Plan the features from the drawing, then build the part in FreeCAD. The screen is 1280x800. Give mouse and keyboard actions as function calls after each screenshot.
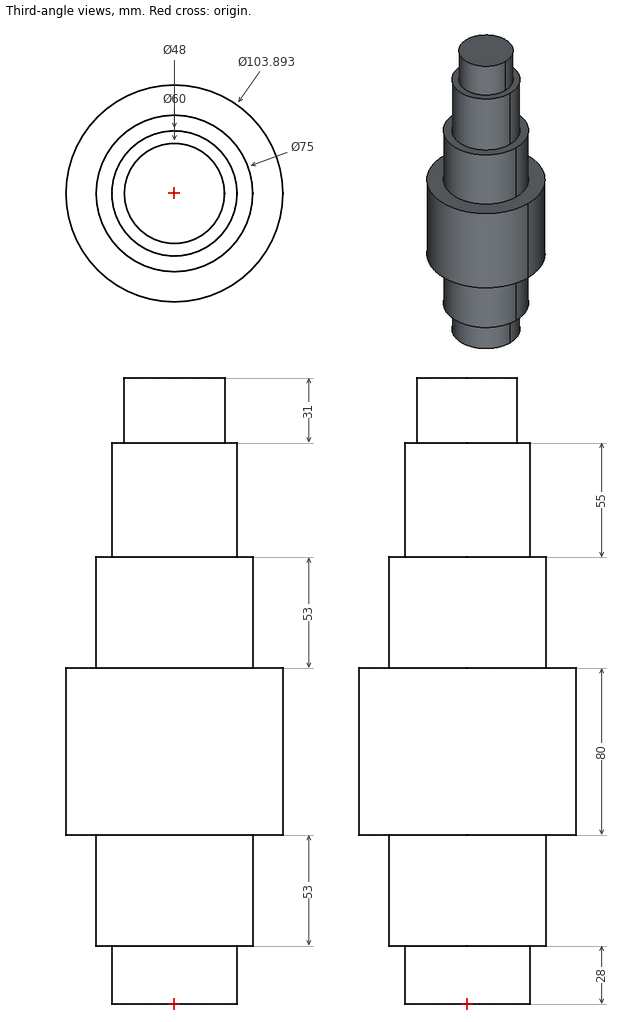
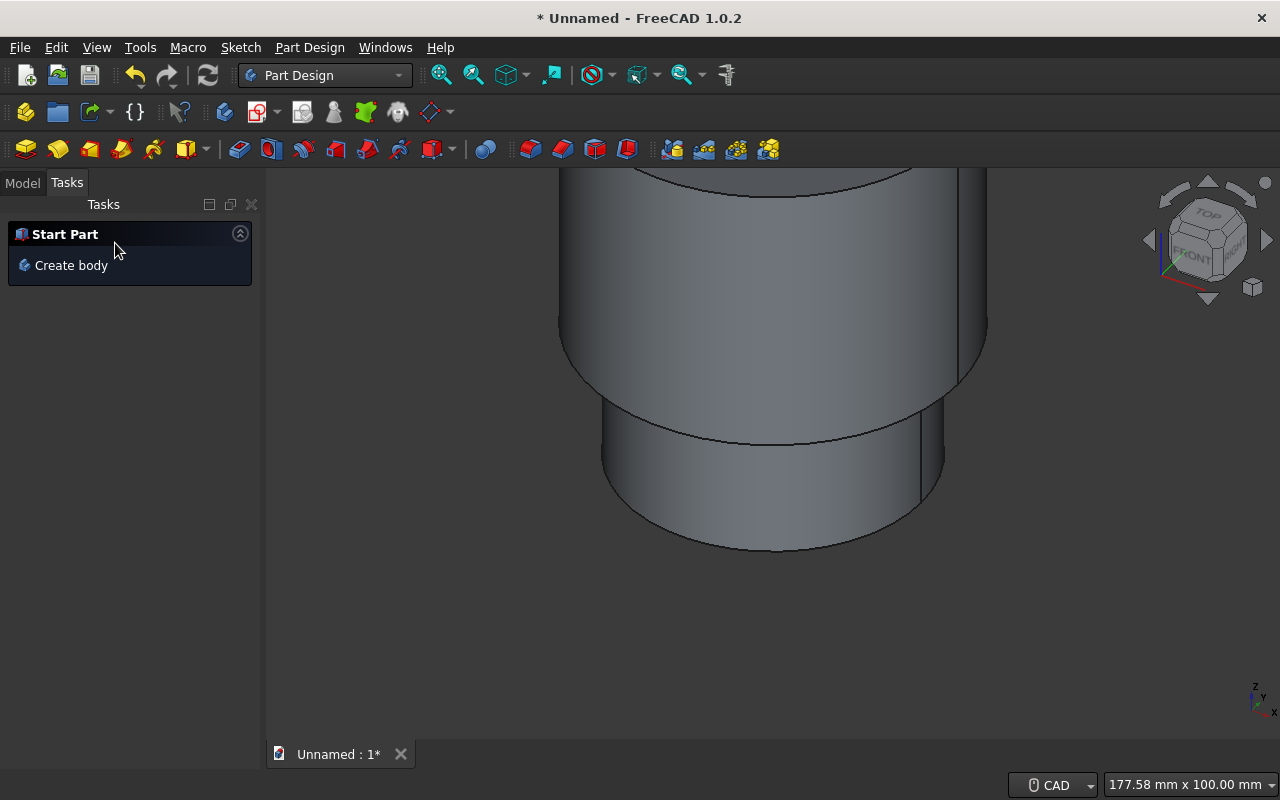
click(442, 76)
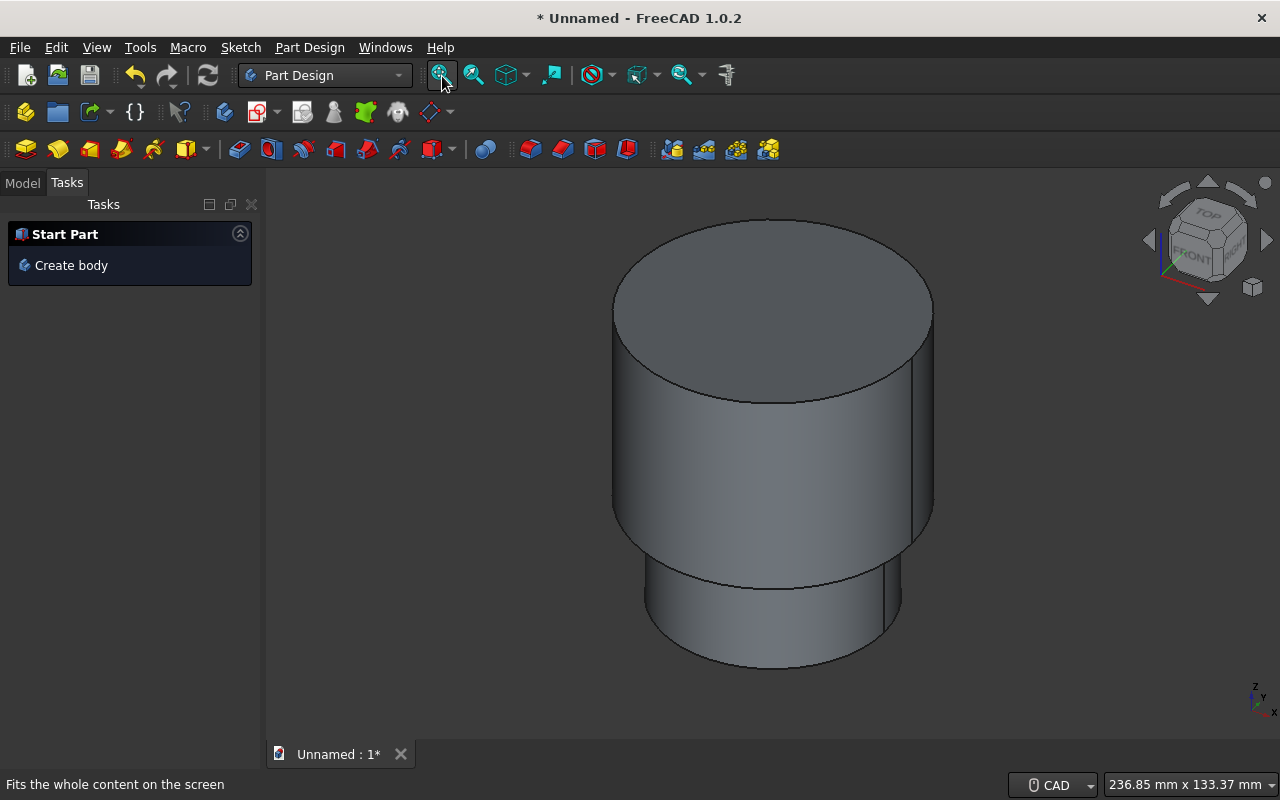
click(773, 310)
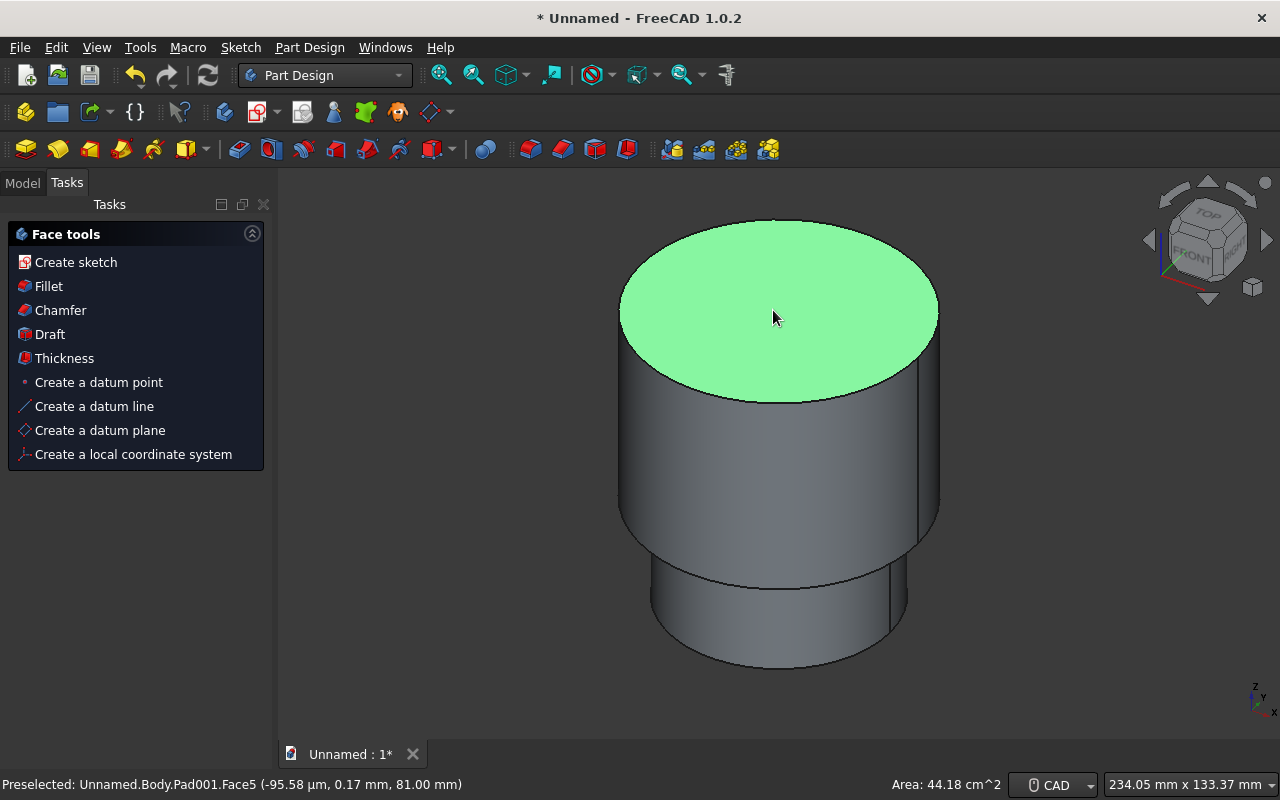
click(258, 112)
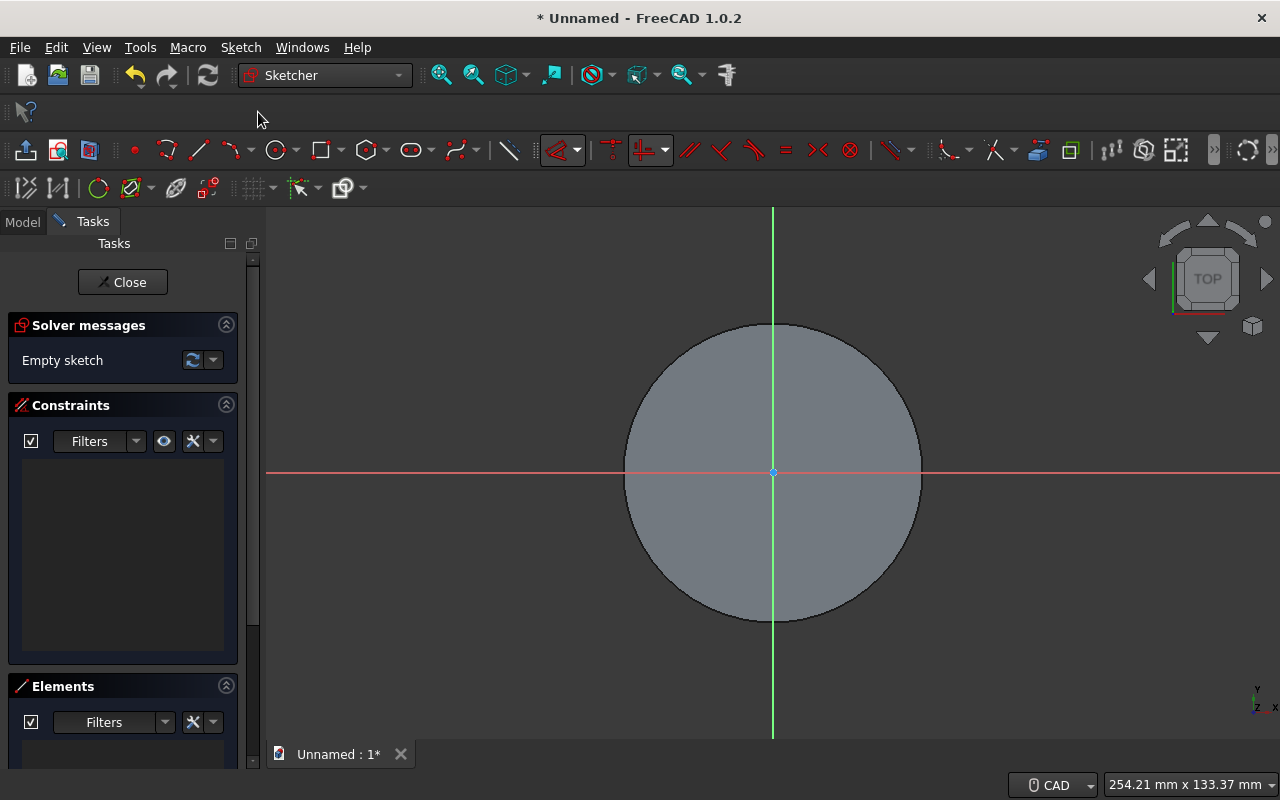
click(276, 150)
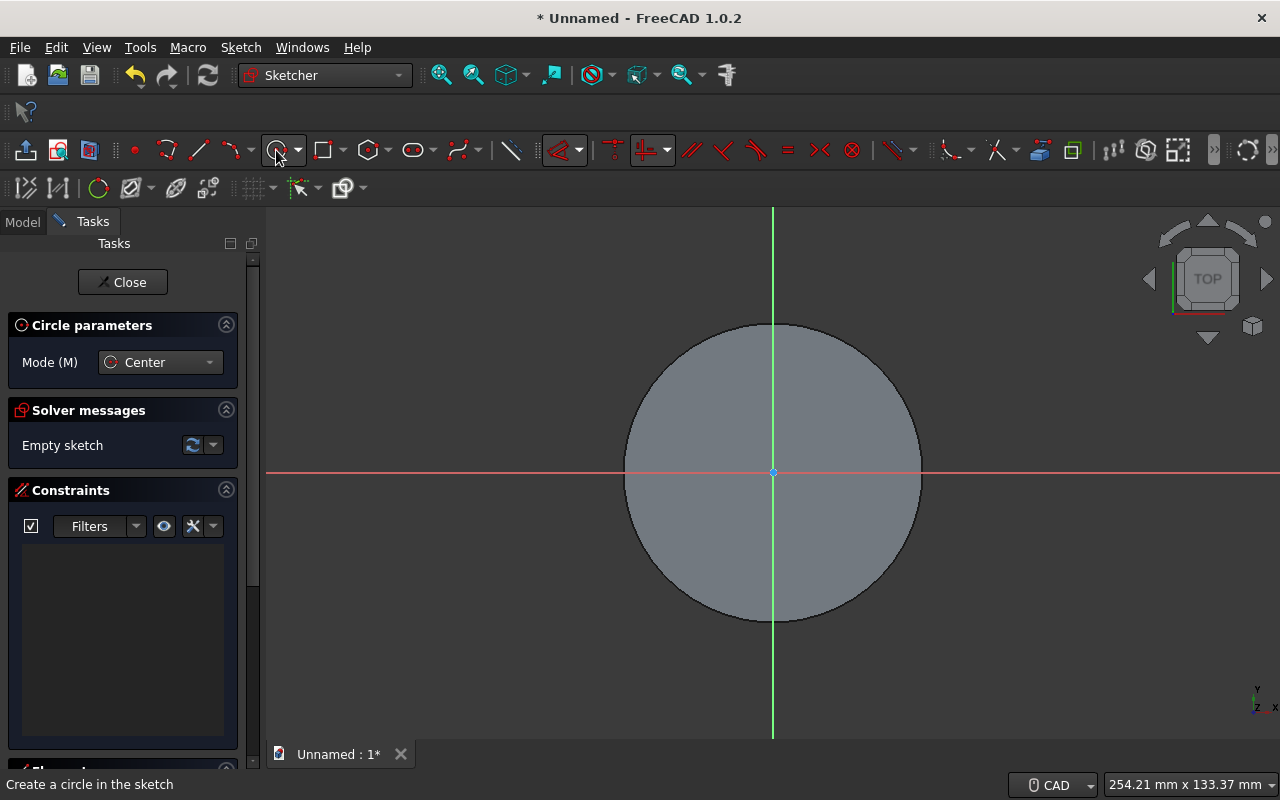
click(773, 473)
move(920, 326)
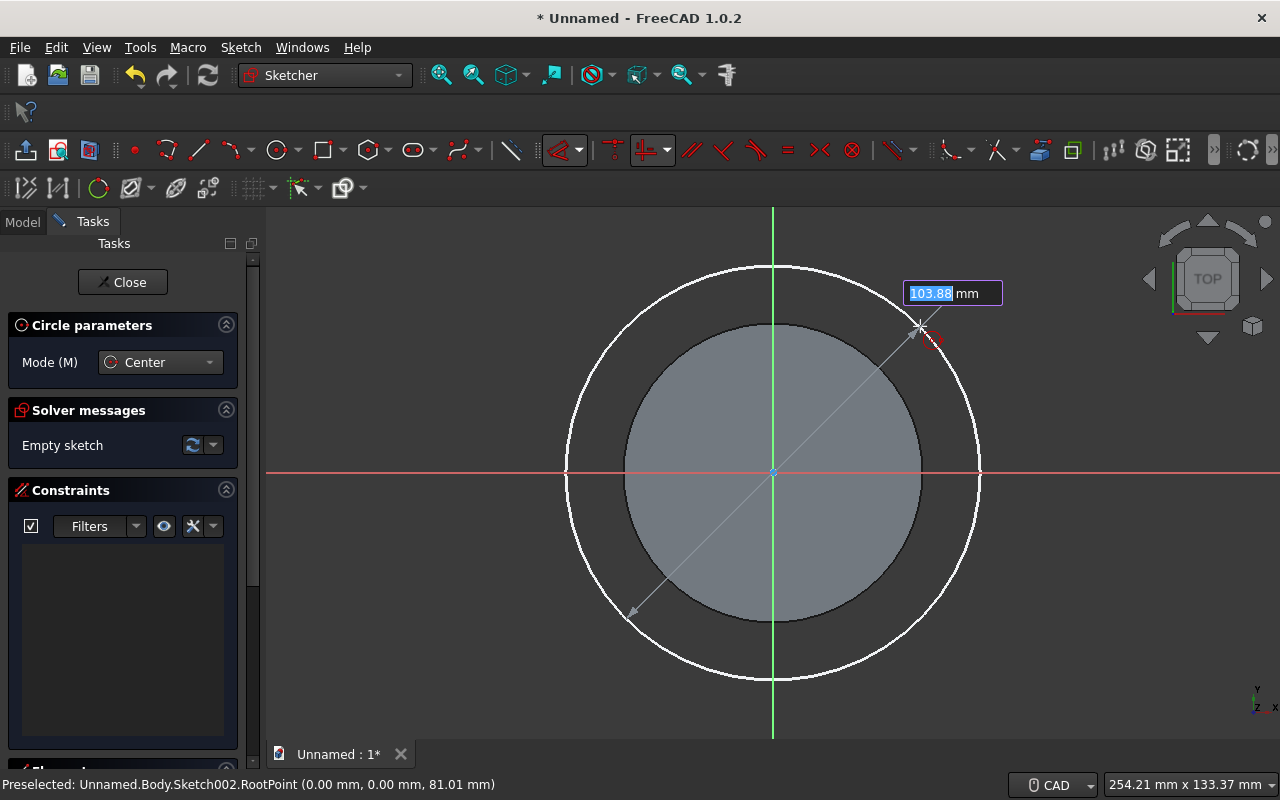
text(103.893)
key(Return)
key(Escape)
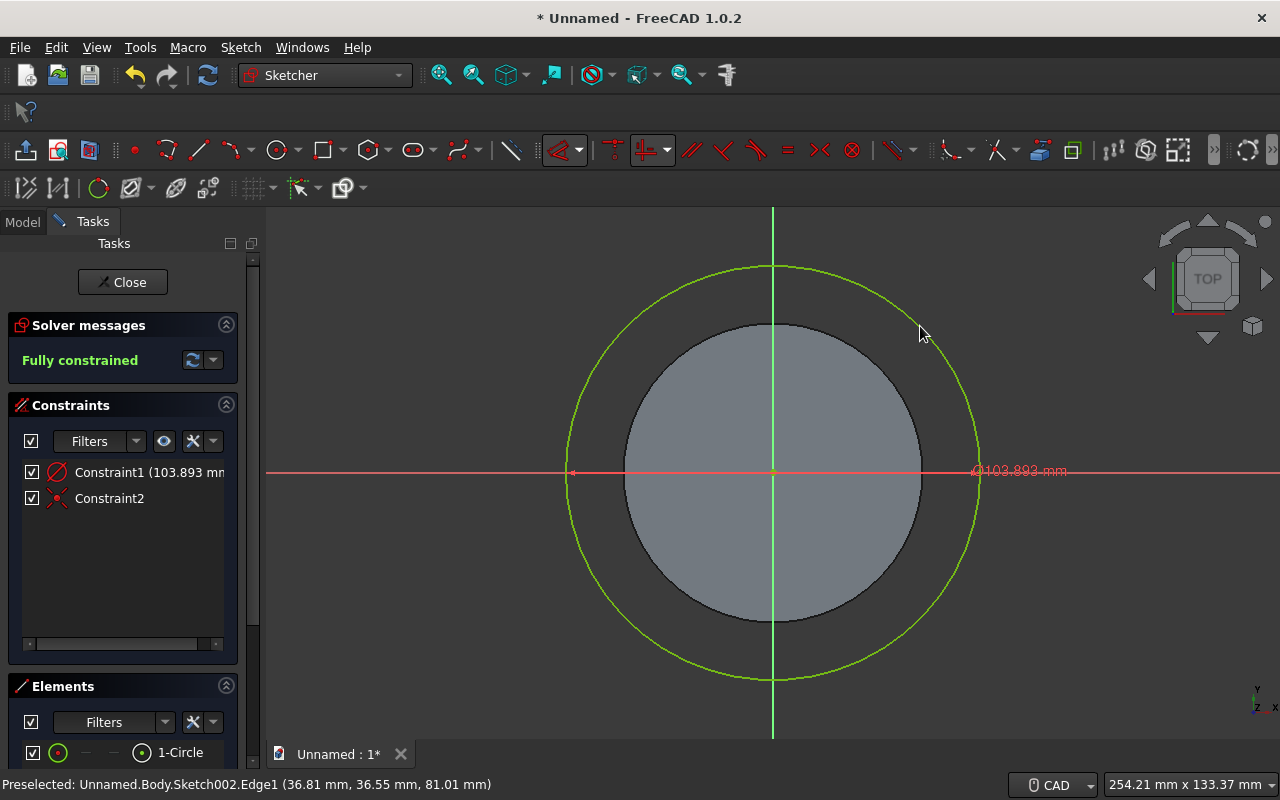
click(123, 282)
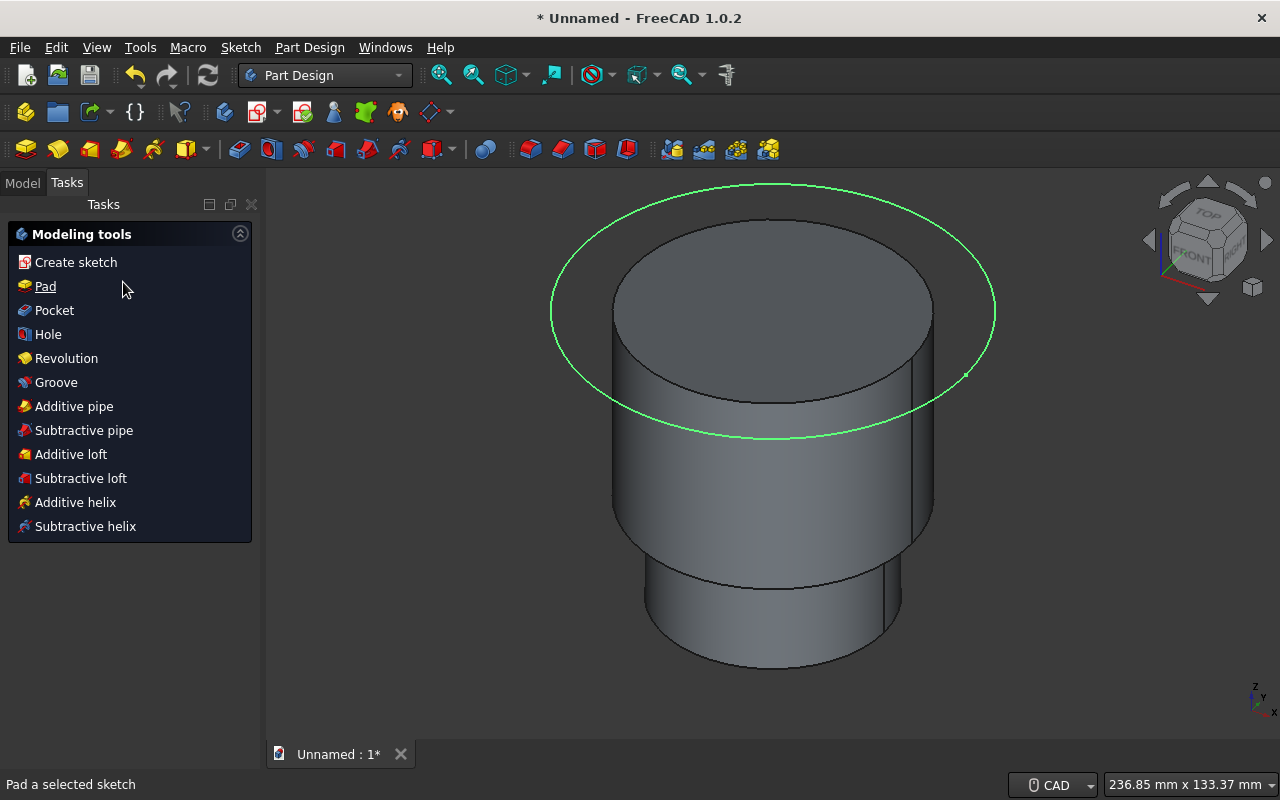
click(26, 150)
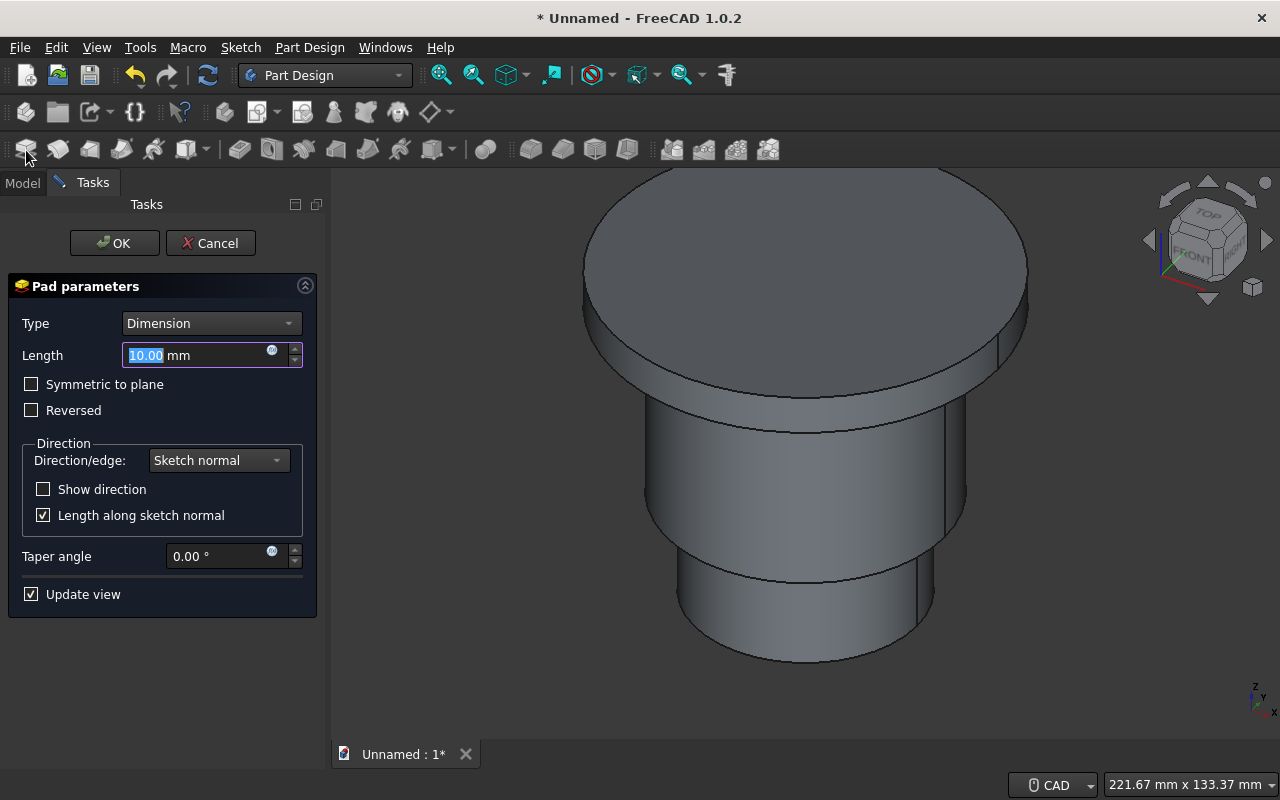
text(80)
key(Tab)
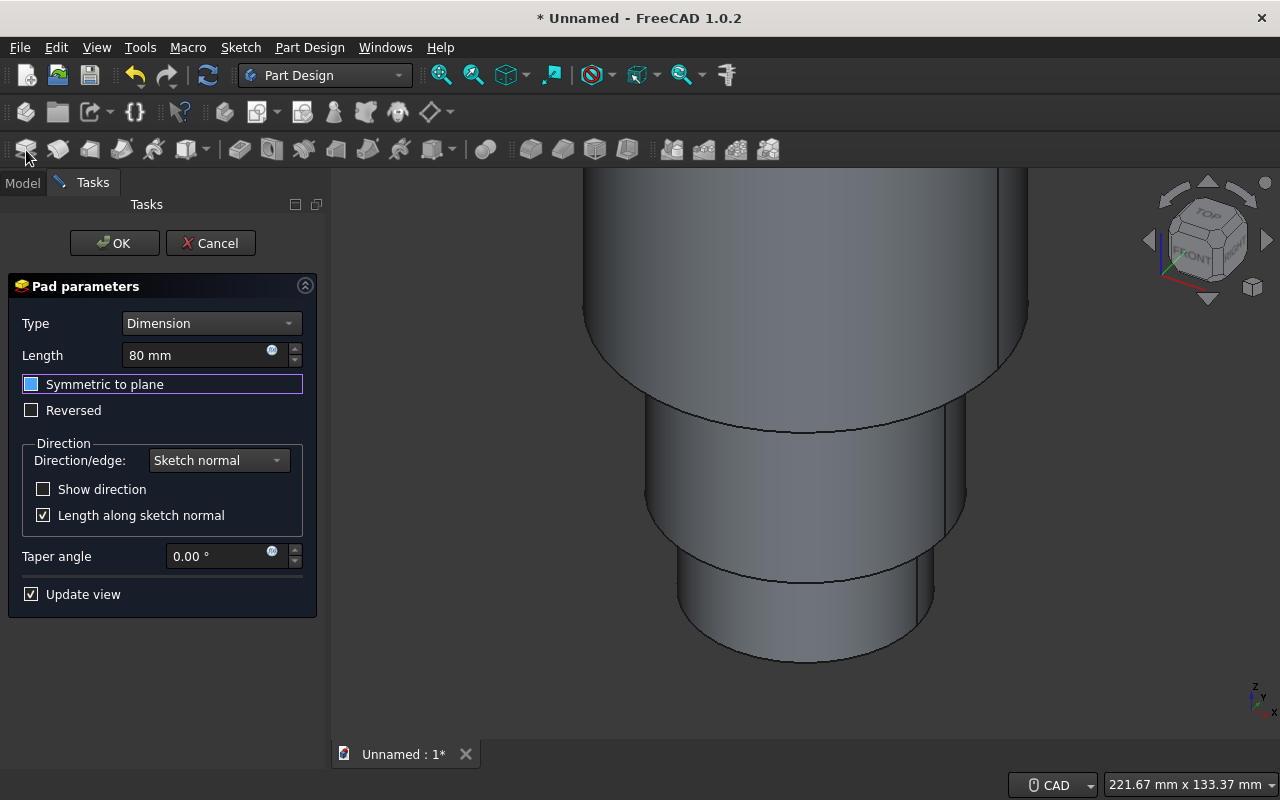
click(115, 243)